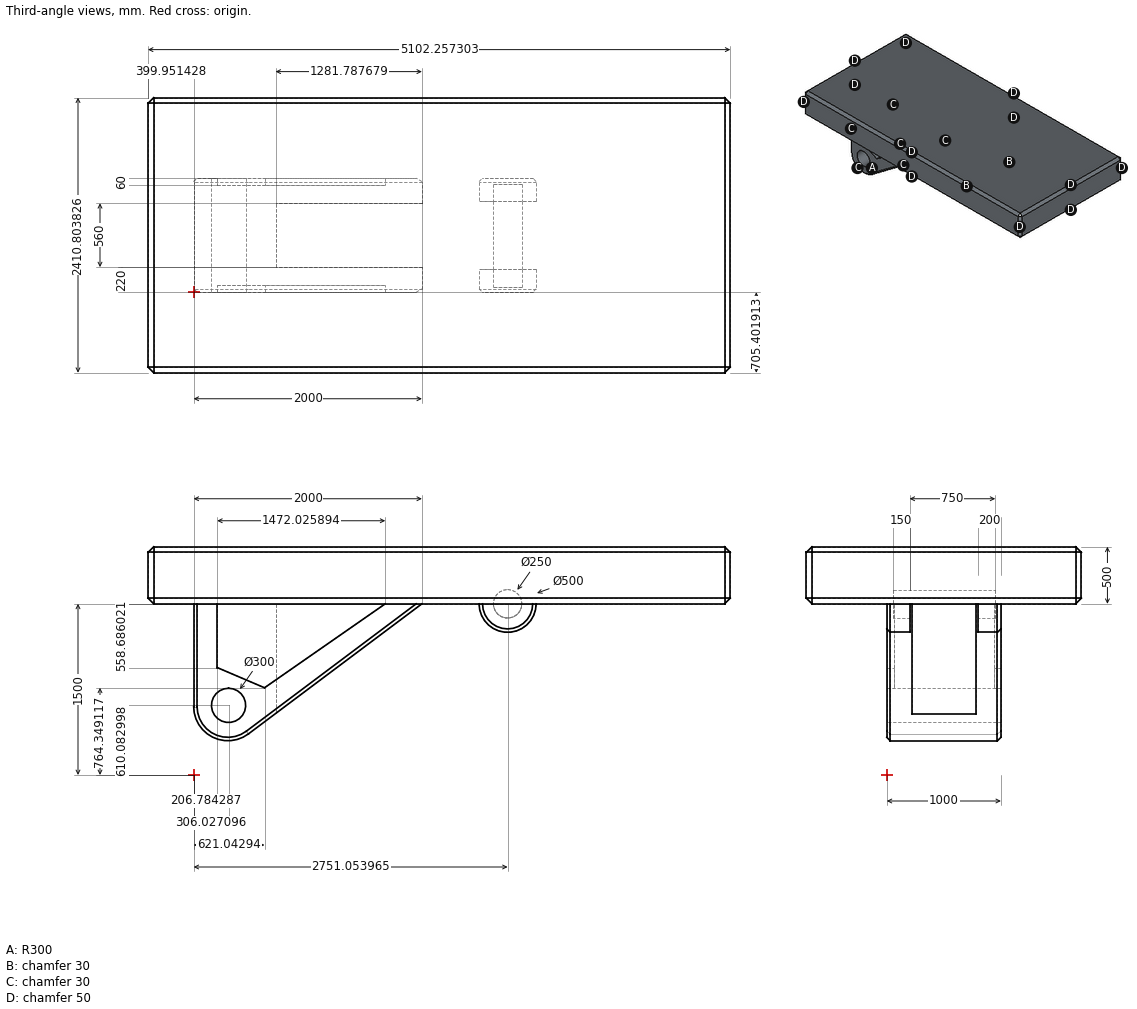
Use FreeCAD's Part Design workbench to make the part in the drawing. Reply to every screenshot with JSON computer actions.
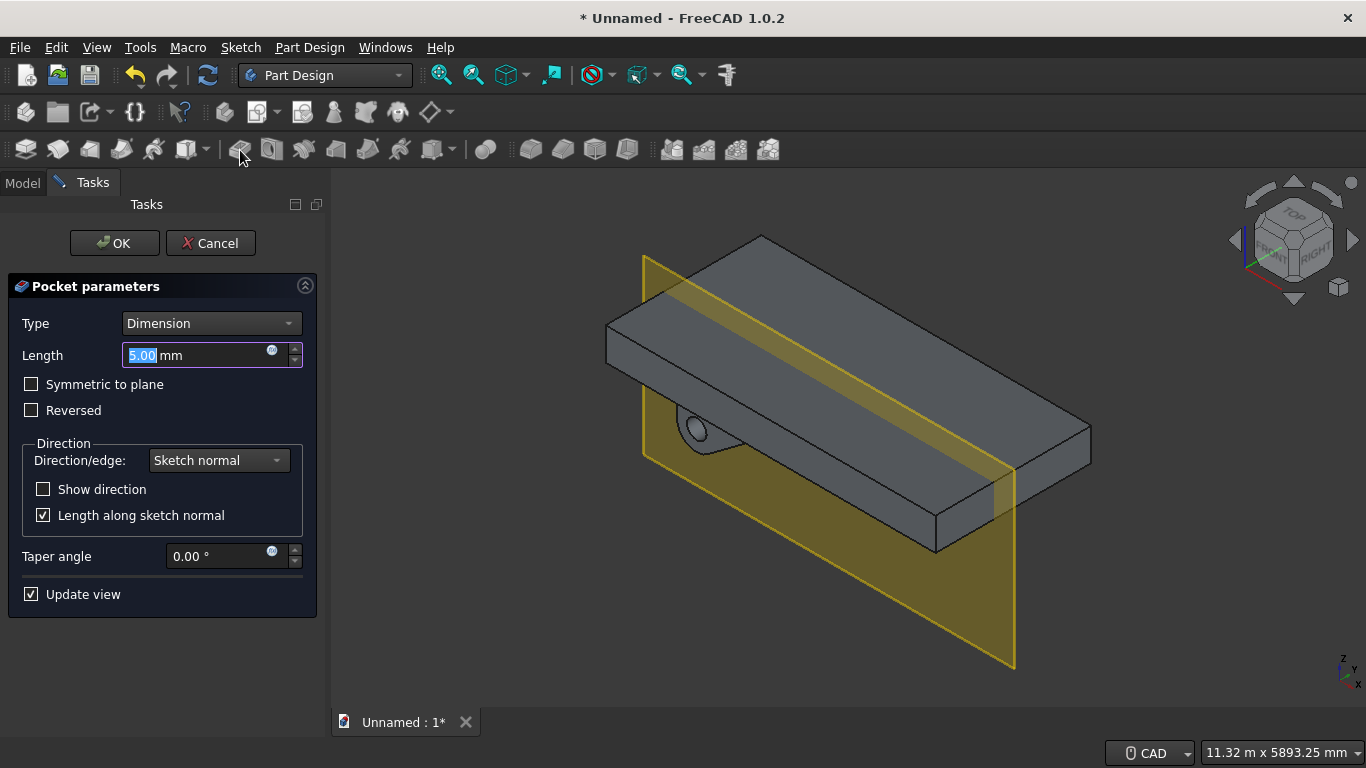
{"action": "left_click", "coordinate": [212, 324]}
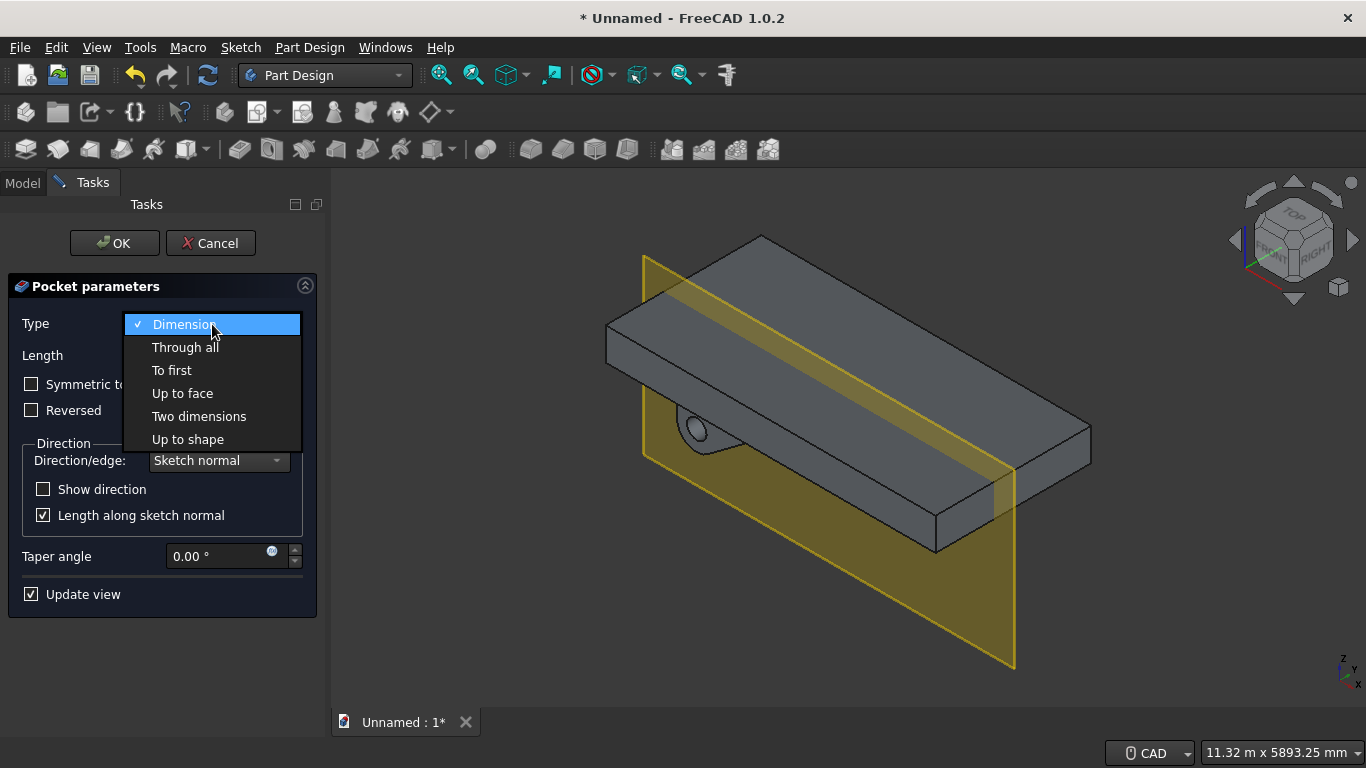
{"action": "left_click", "coordinate": [212, 416]}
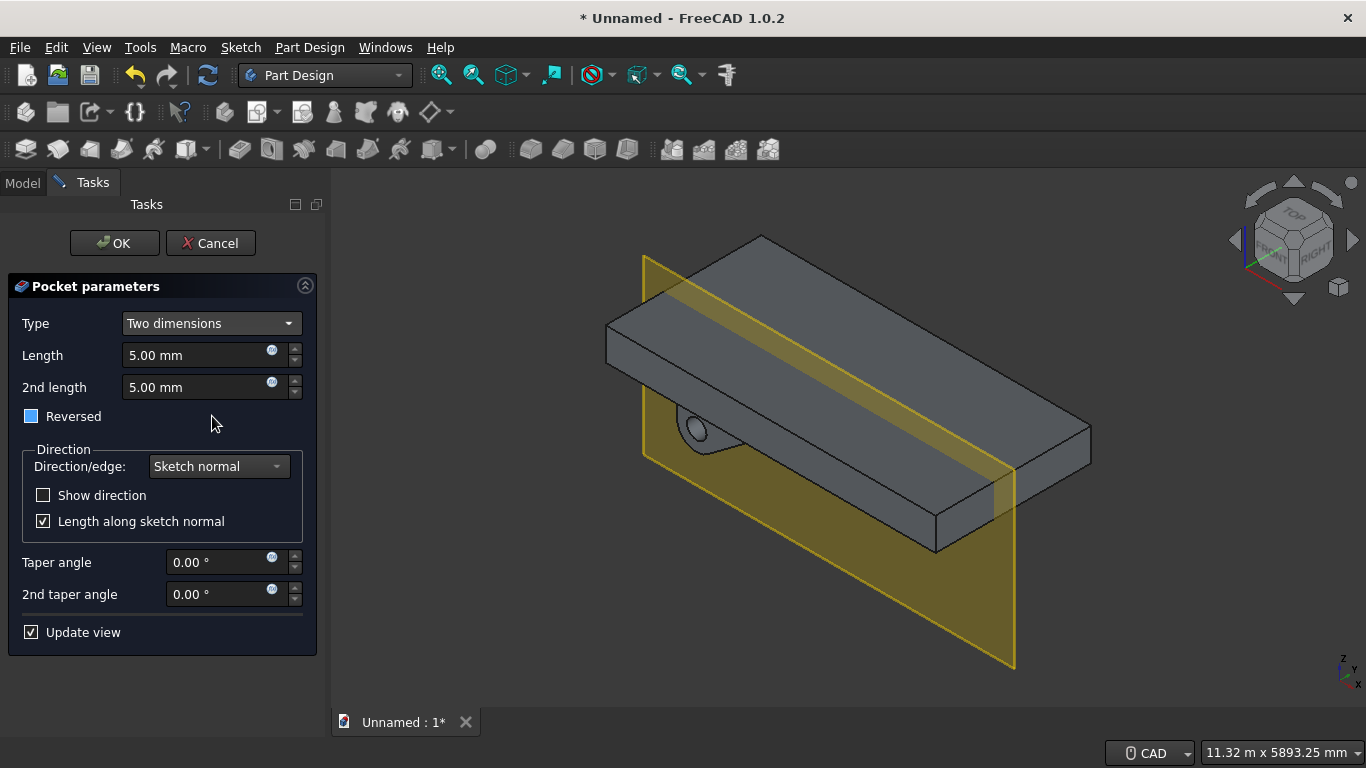
{"action": "triple_click", "coordinate": [204, 355]}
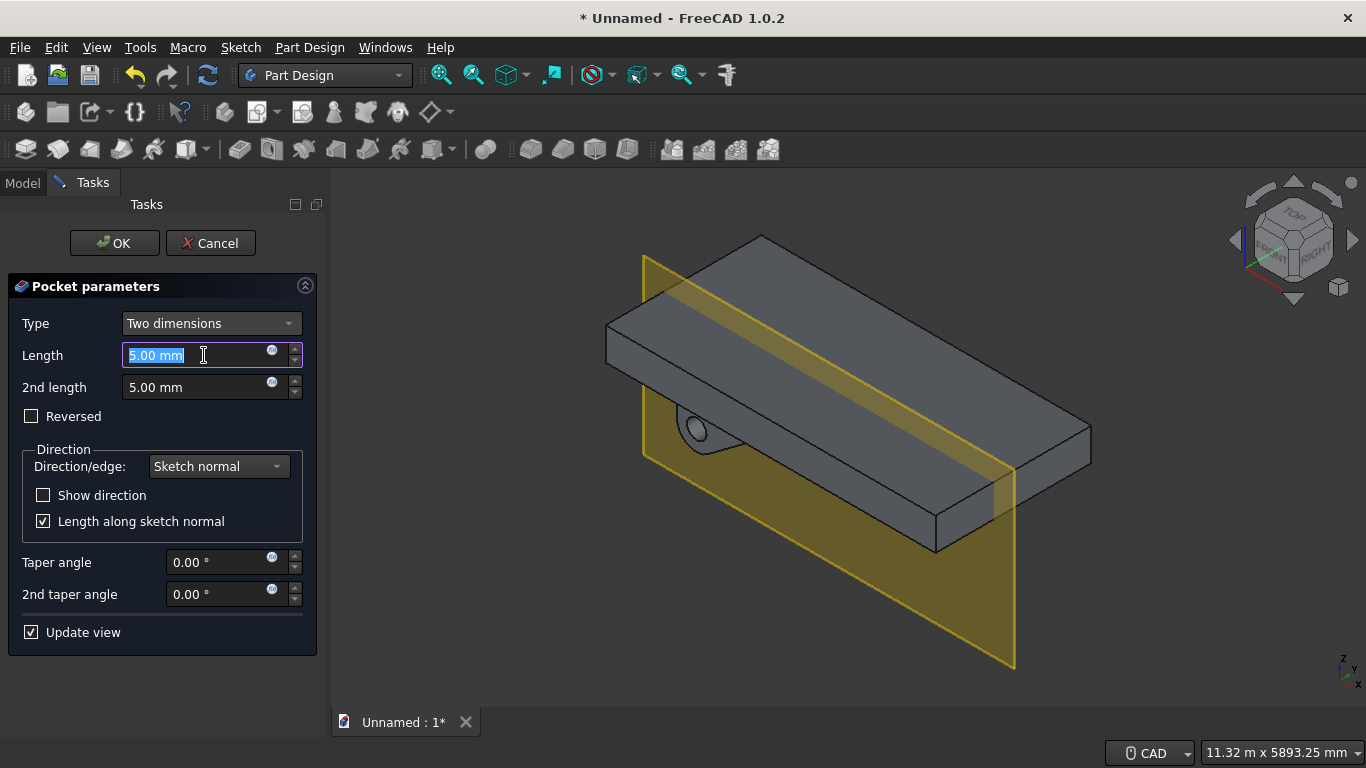
{"action": "type", "text": "750"}
{"action": "key", "text": "Tab"}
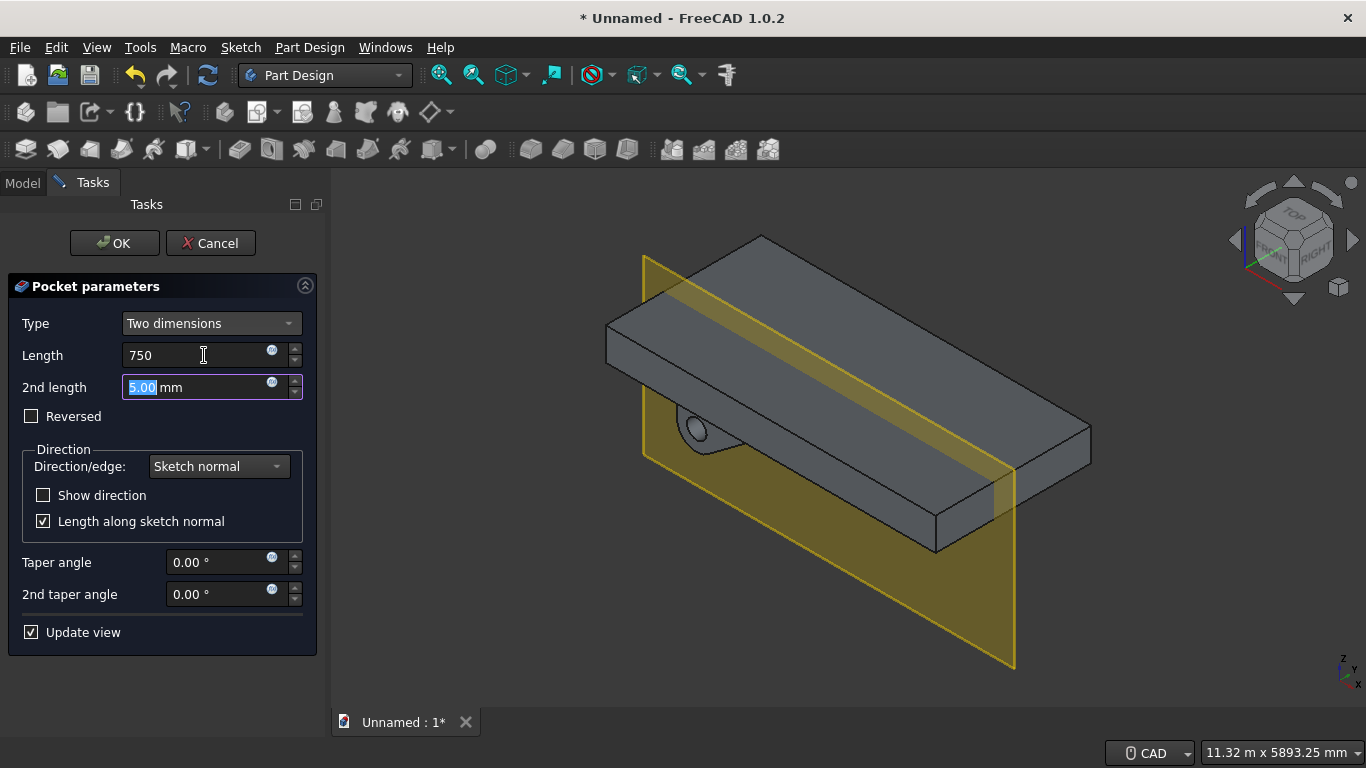
{"action": "type", "text": "150"}
{"action": "key", "text": "Tab"}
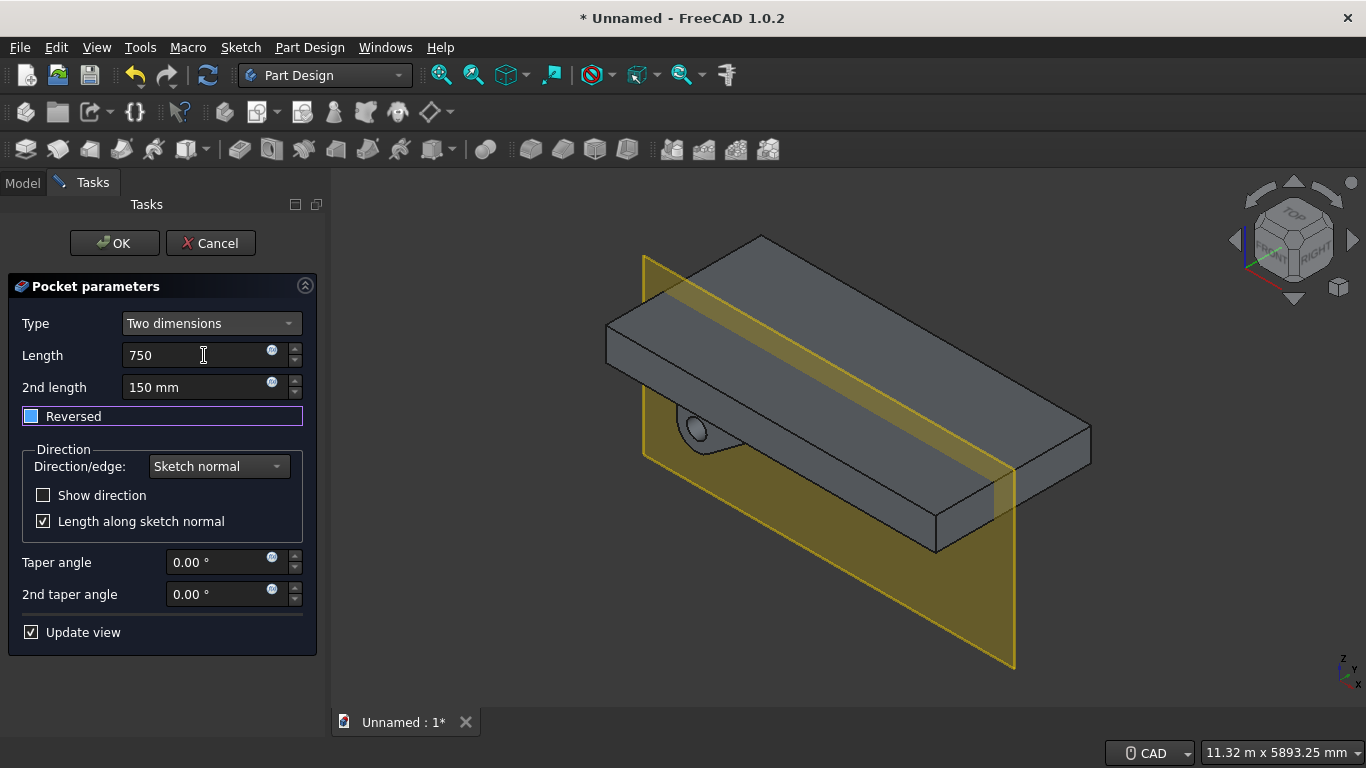
{"action": "left_click", "coordinate": [115, 243]}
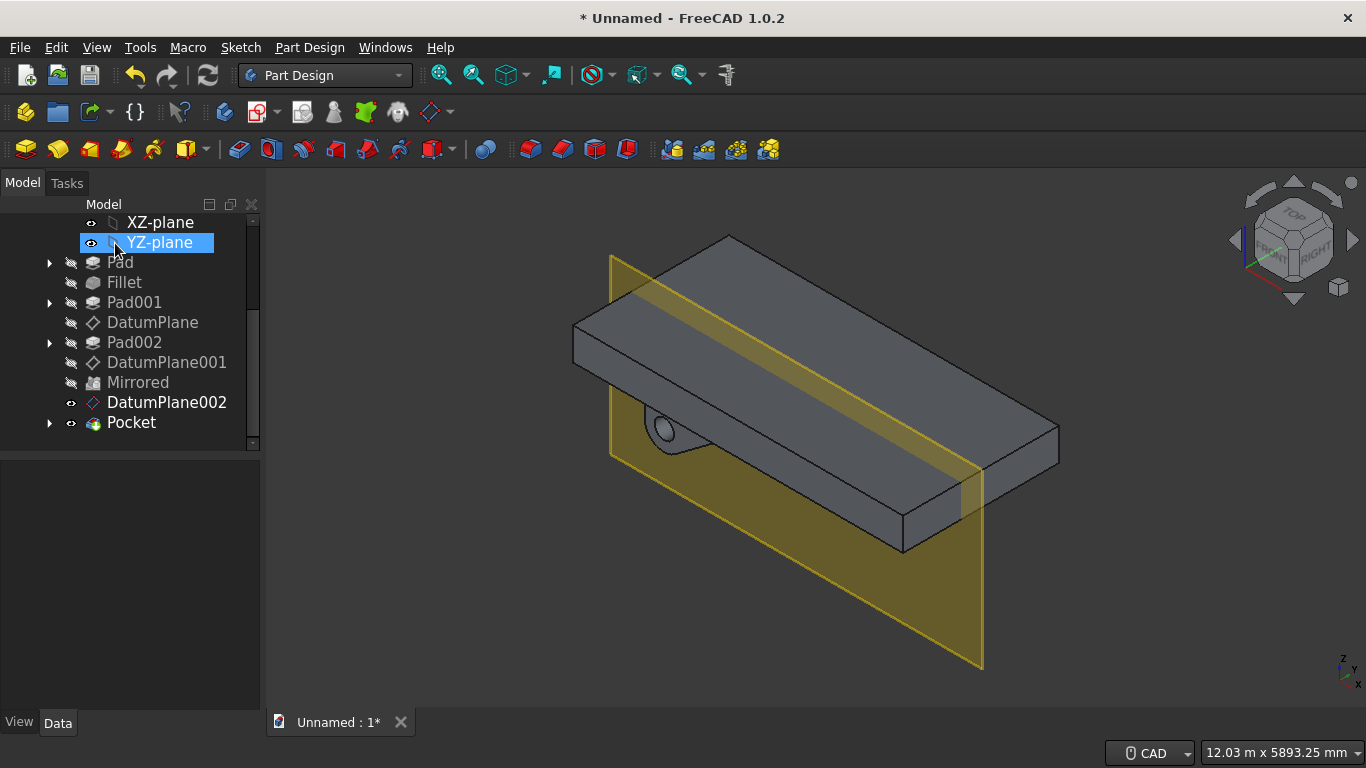
{"action": "left_click", "coordinate": [116, 403]}
{"action": "key", "text": "space"}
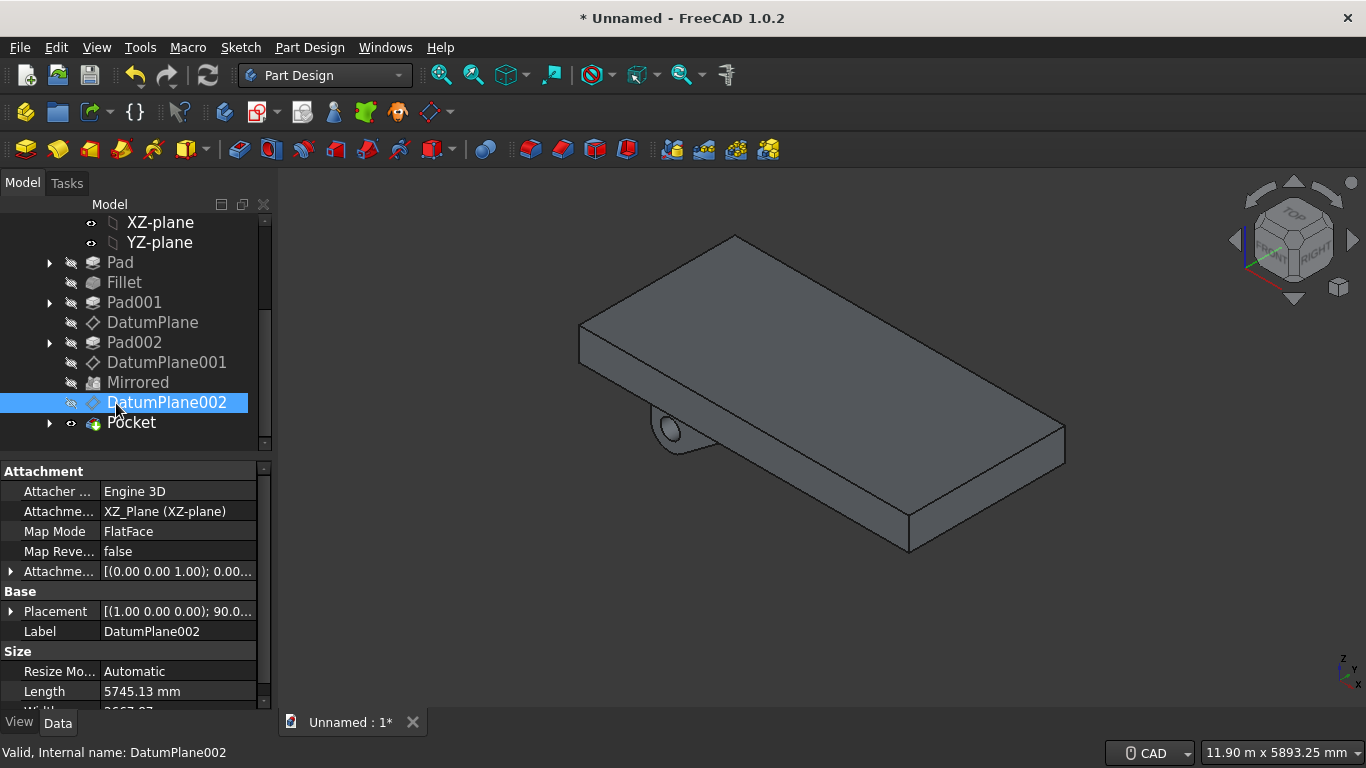
{"action": "key", "text": "2"}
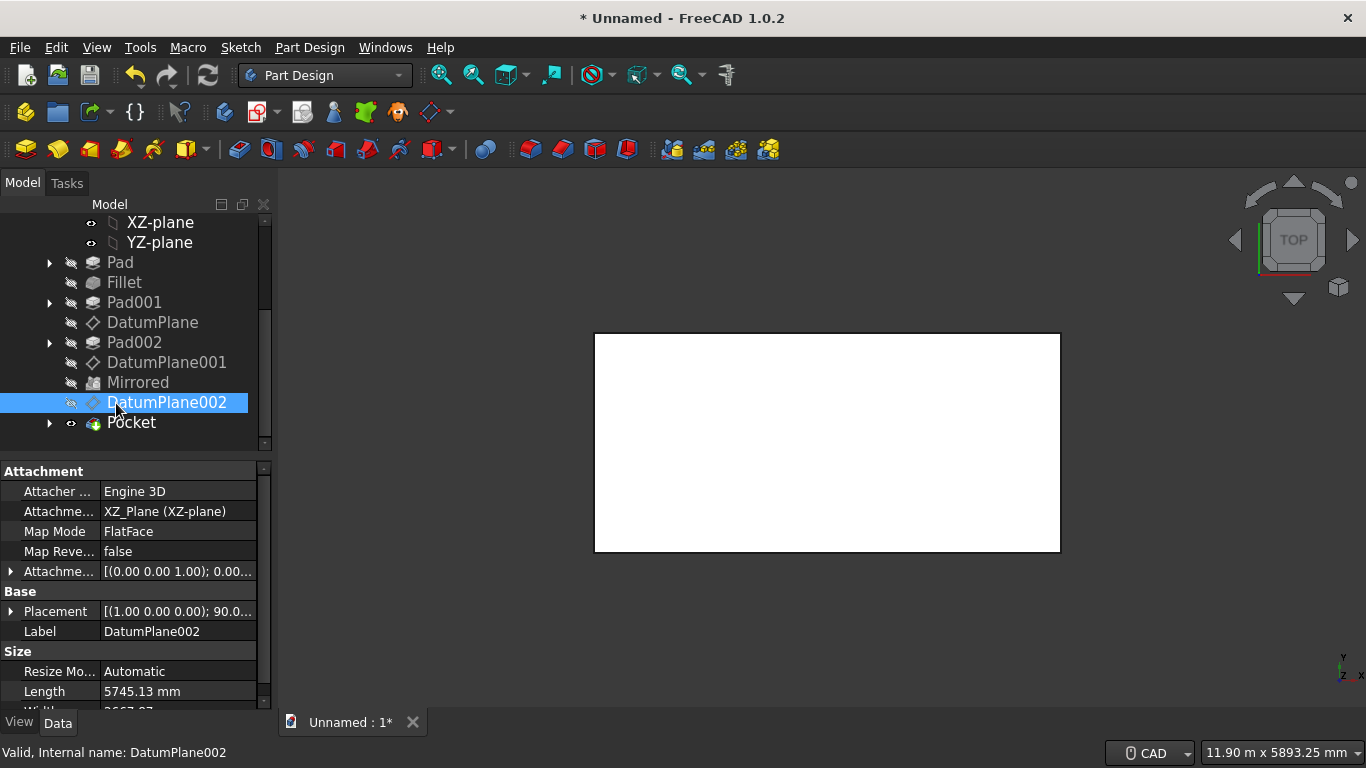
{"action": "left_click", "coordinate": [442, 76]}